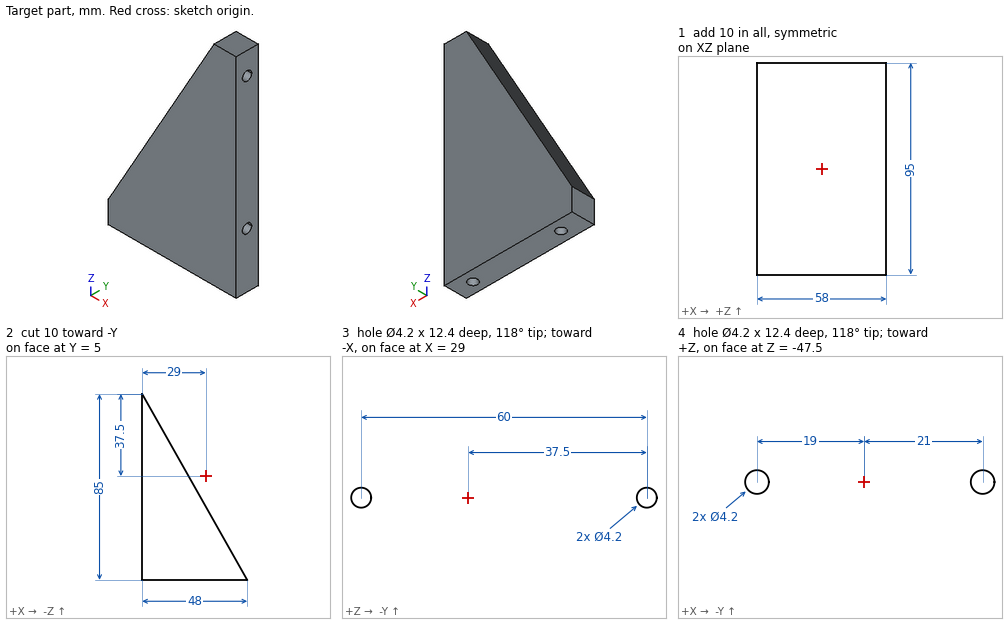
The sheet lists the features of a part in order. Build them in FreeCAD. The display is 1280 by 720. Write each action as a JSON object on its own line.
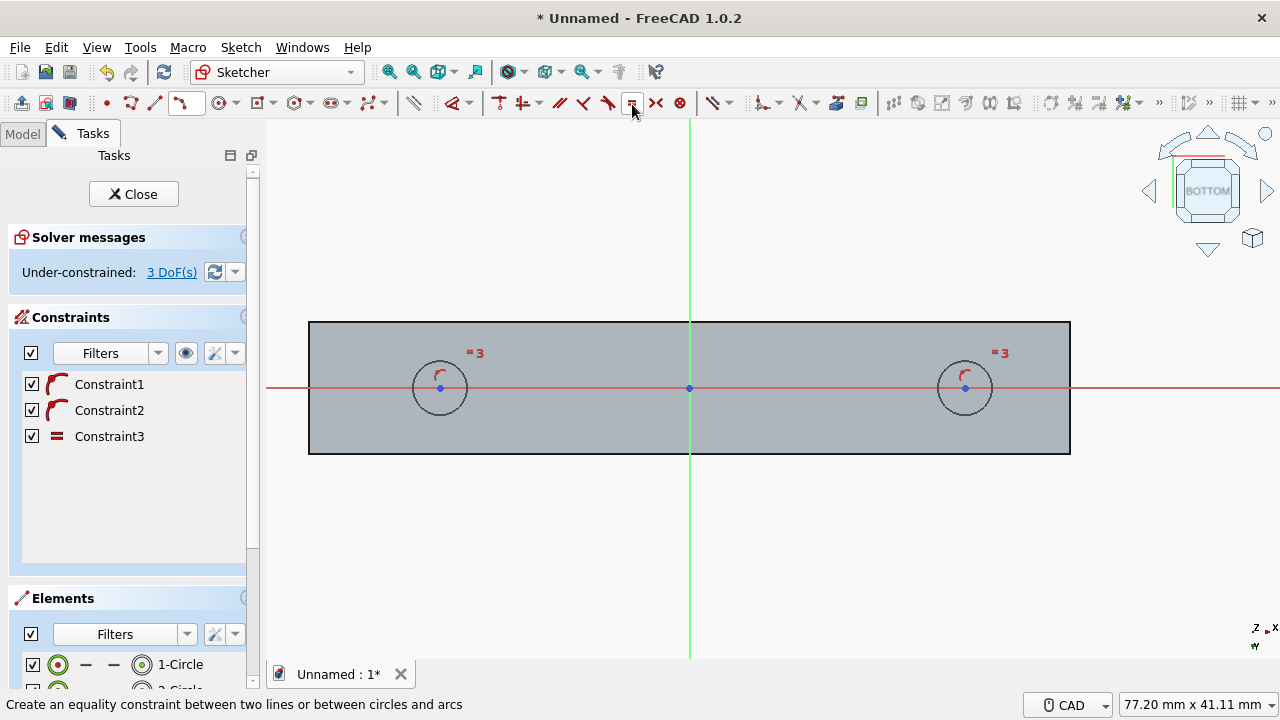
{"action": "left_click", "coordinate": [452, 104]}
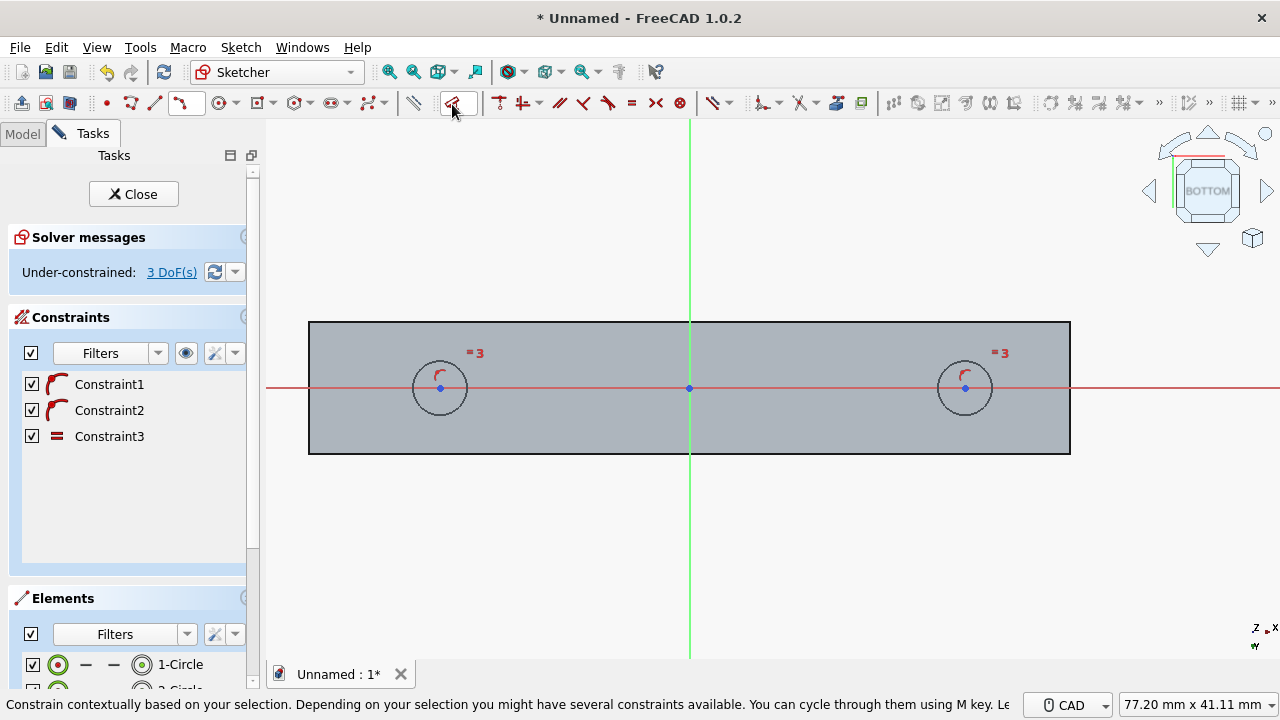
{"action": "left_click", "coordinate": [459, 369]}
{"action": "left_click", "coordinate": [482, 346]}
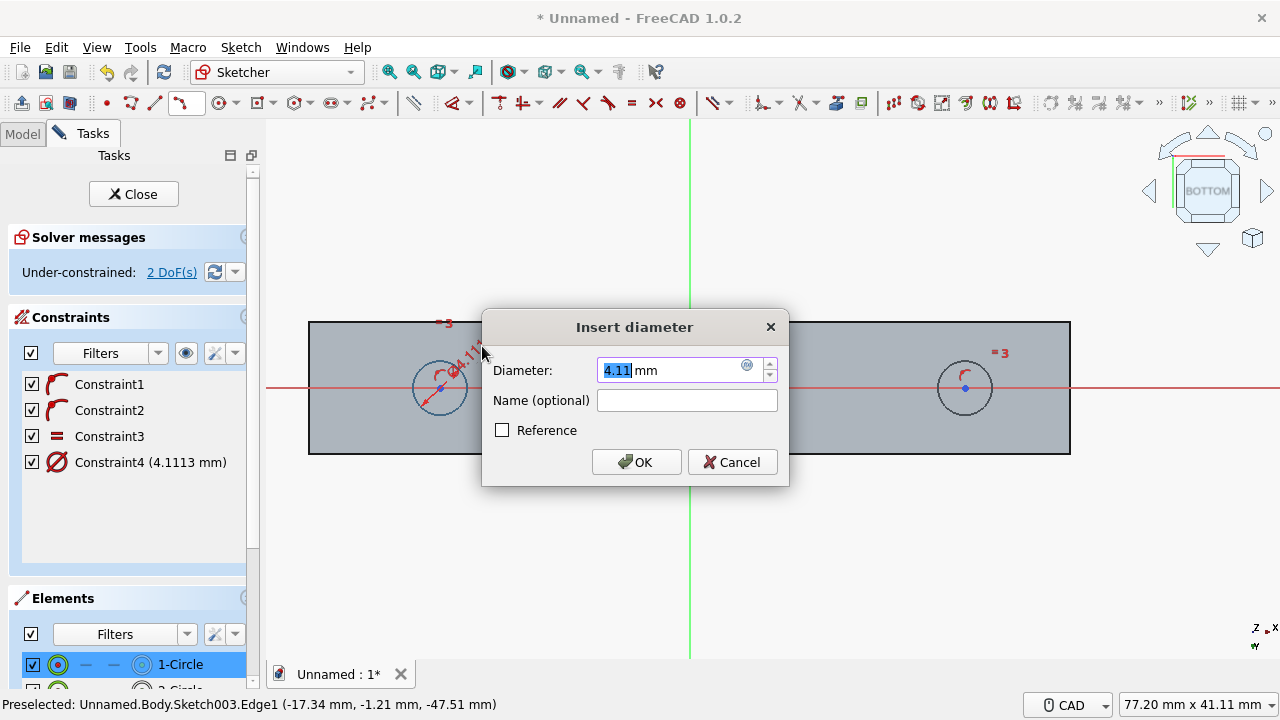
{"action": "type", "text": "4.2"}
{"action": "key", "text": "Return"}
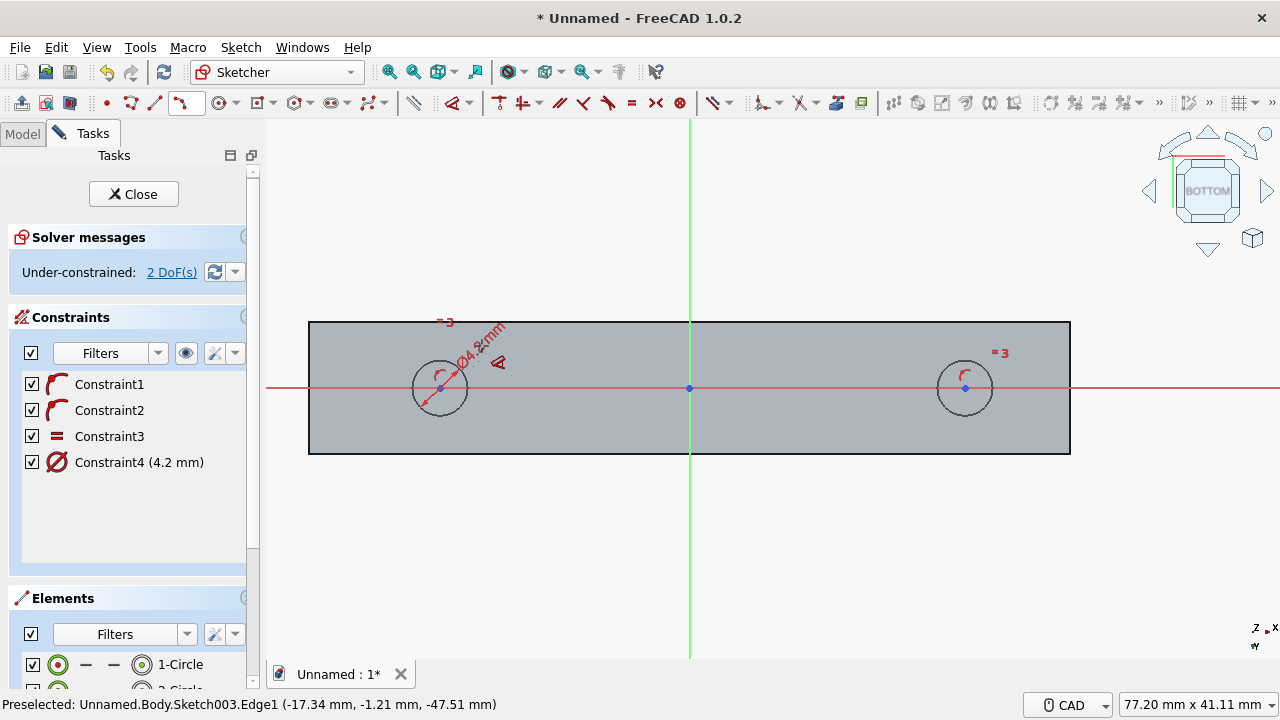
{"action": "left_click", "coordinate": [440, 388]}
{"action": "left_click", "coordinate": [565, 422]}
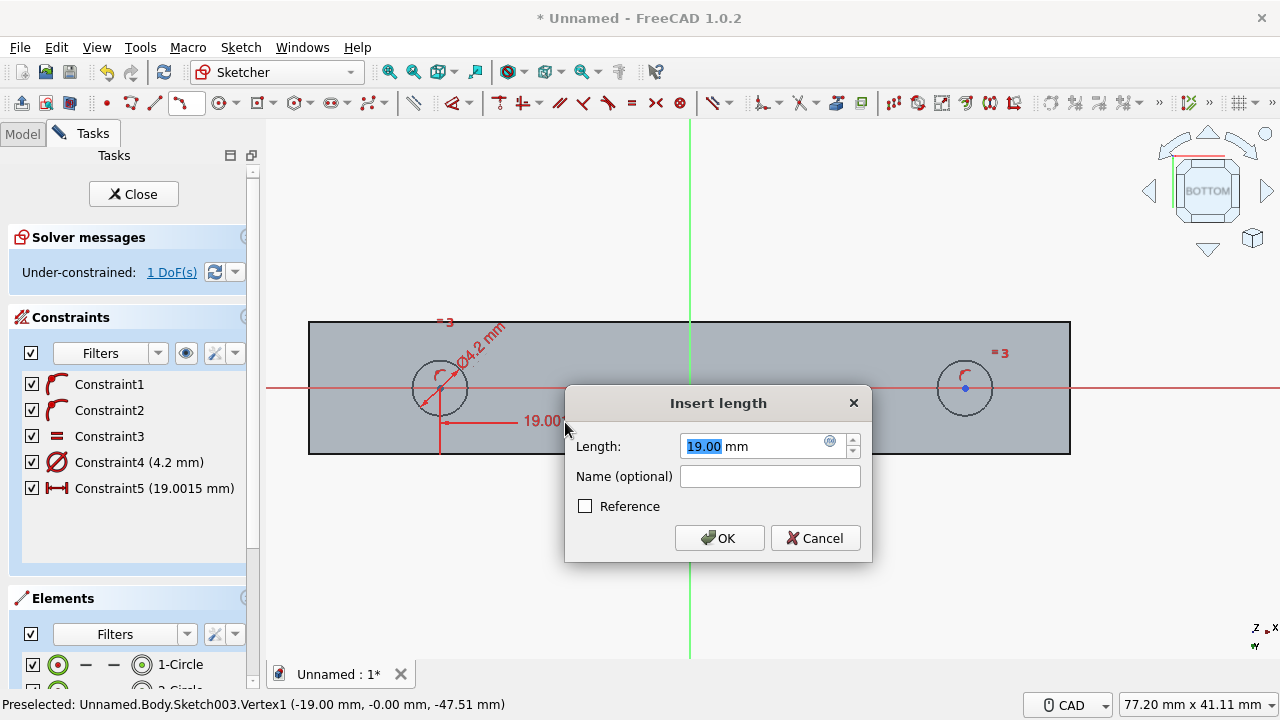
{"action": "type", "text": "19"}
{"action": "key", "text": "Return"}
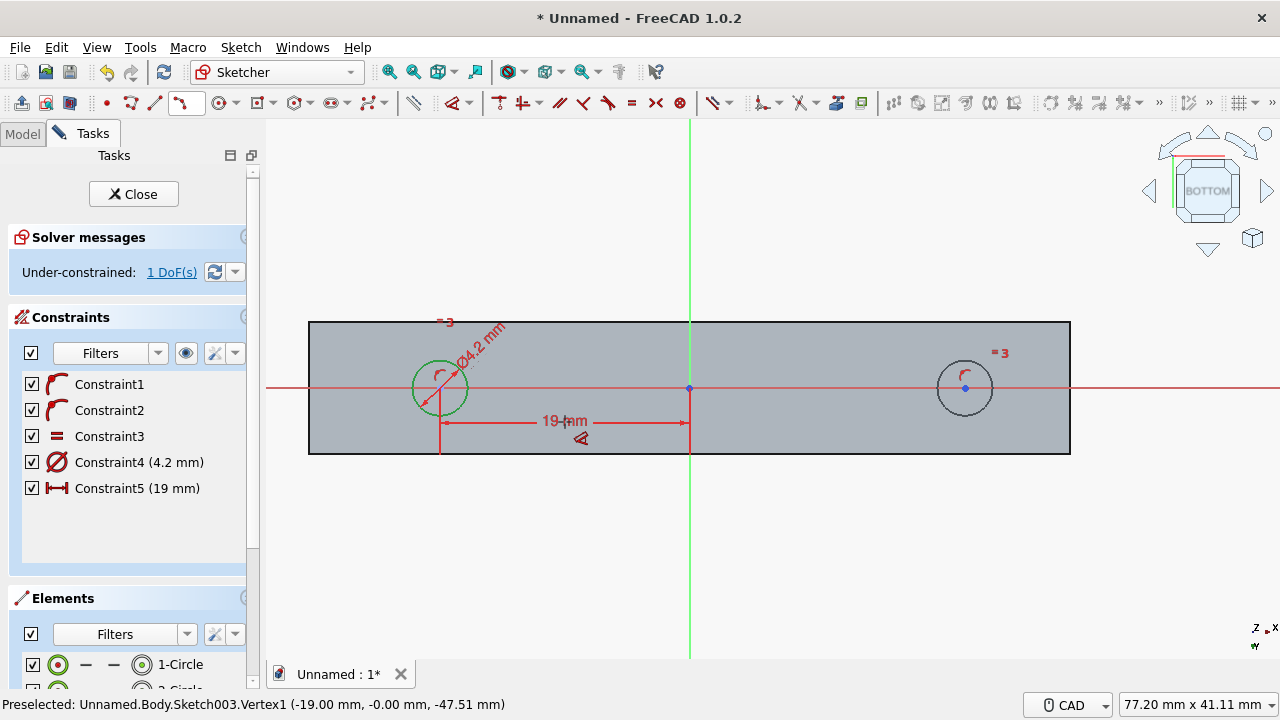
{"action": "left_click", "coordinate": [965, 388]}
{"action": "left_click", "coordinate": [827, 422]}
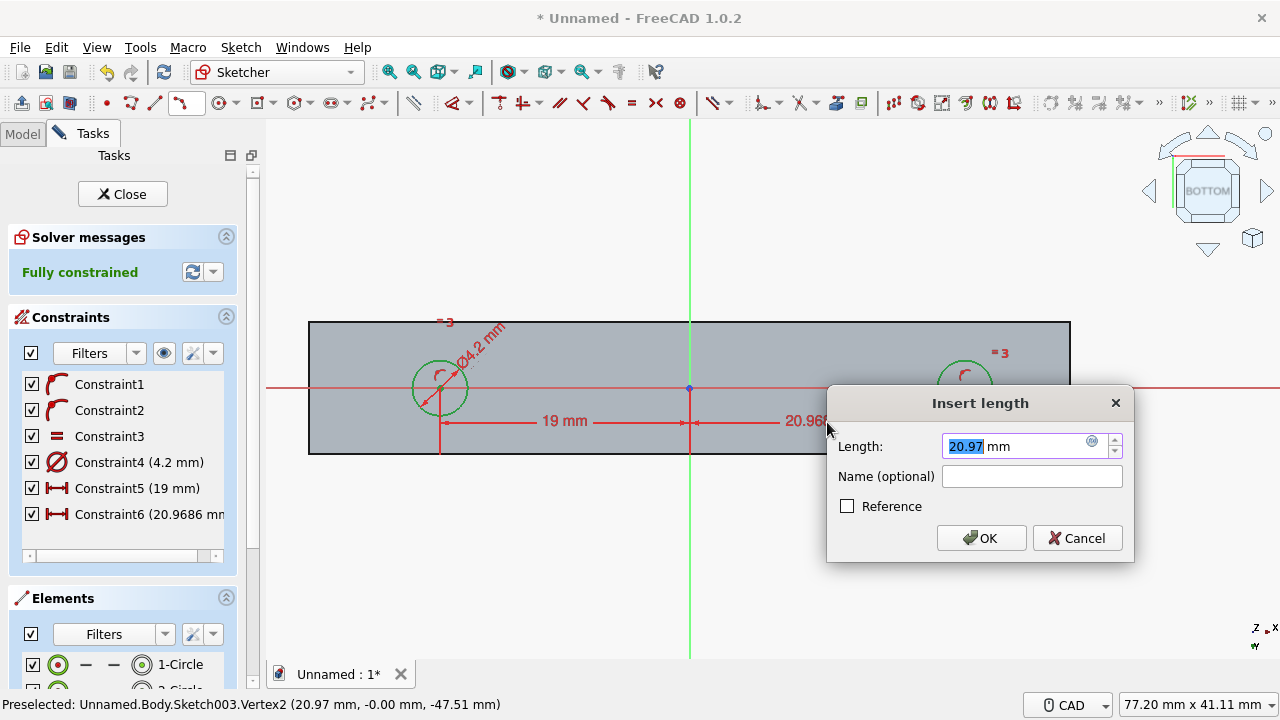
{"action": "type", "text": "21"}
{"action": "key", "text": "Return"}
{"action": "key", "text": "Escape"}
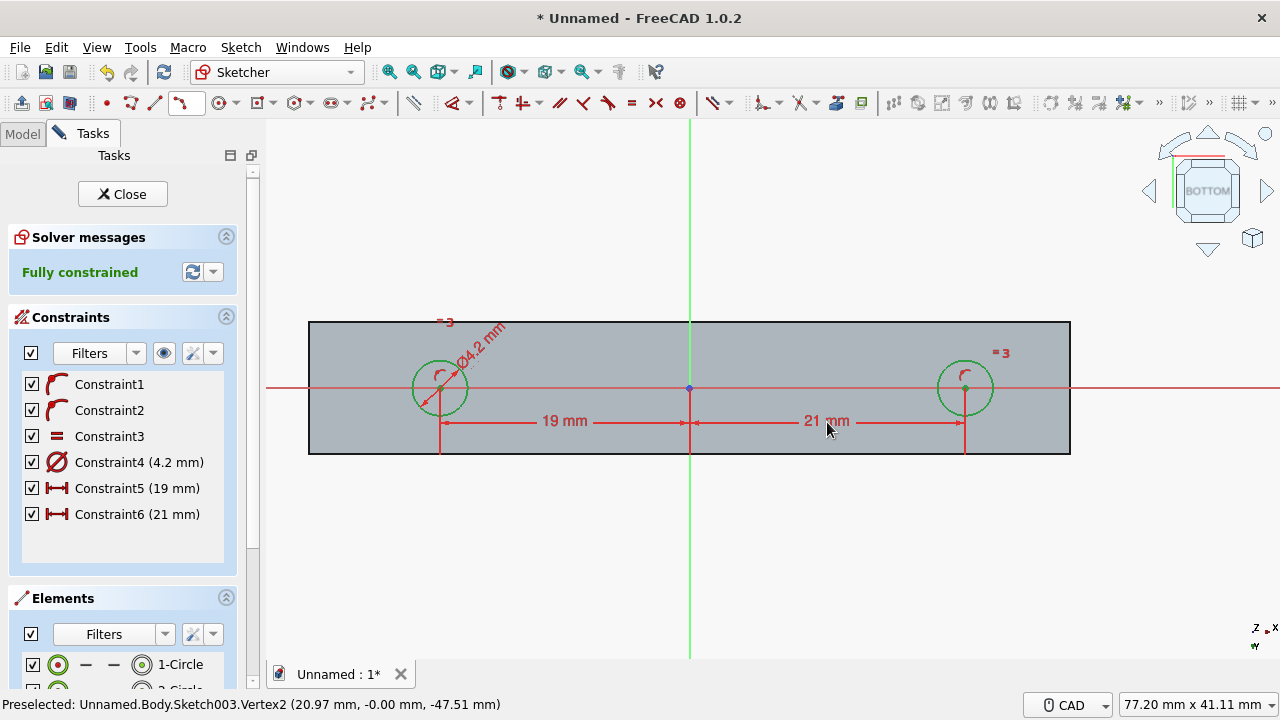
{"action": "left_click", "coordinate": [123, 194]}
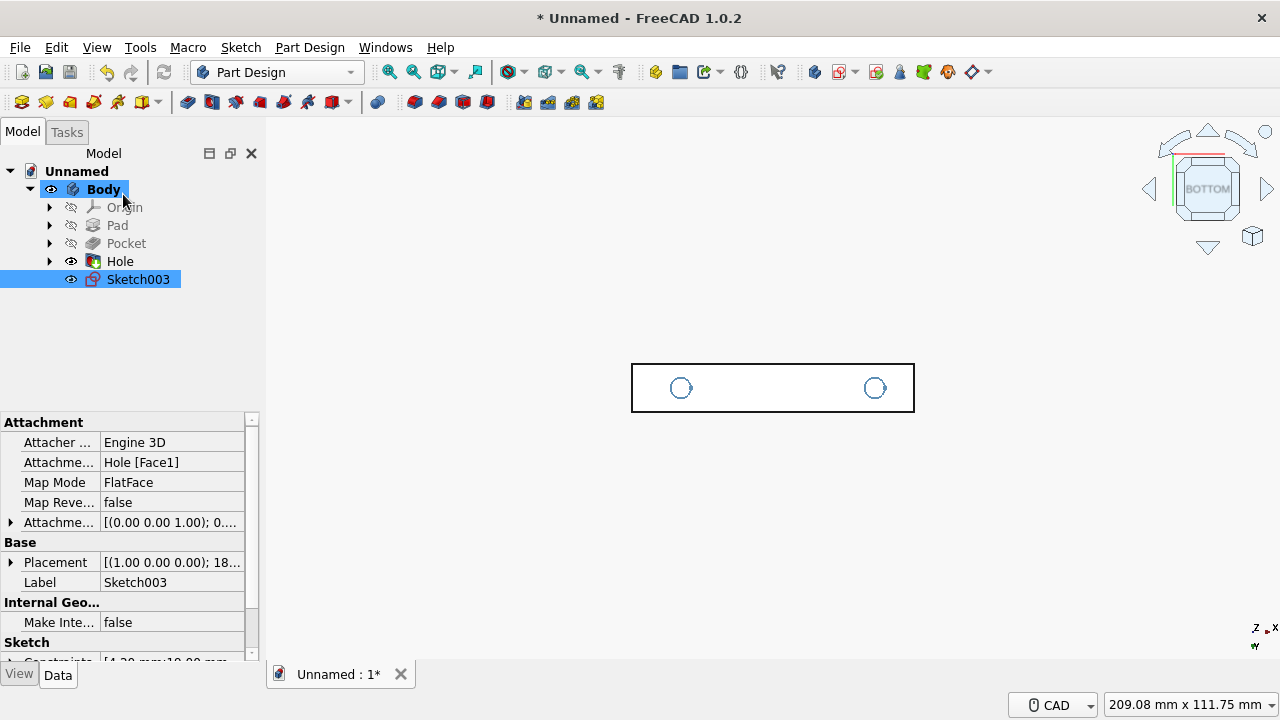
{"action": "left_click", "coordinate": [212, 102]}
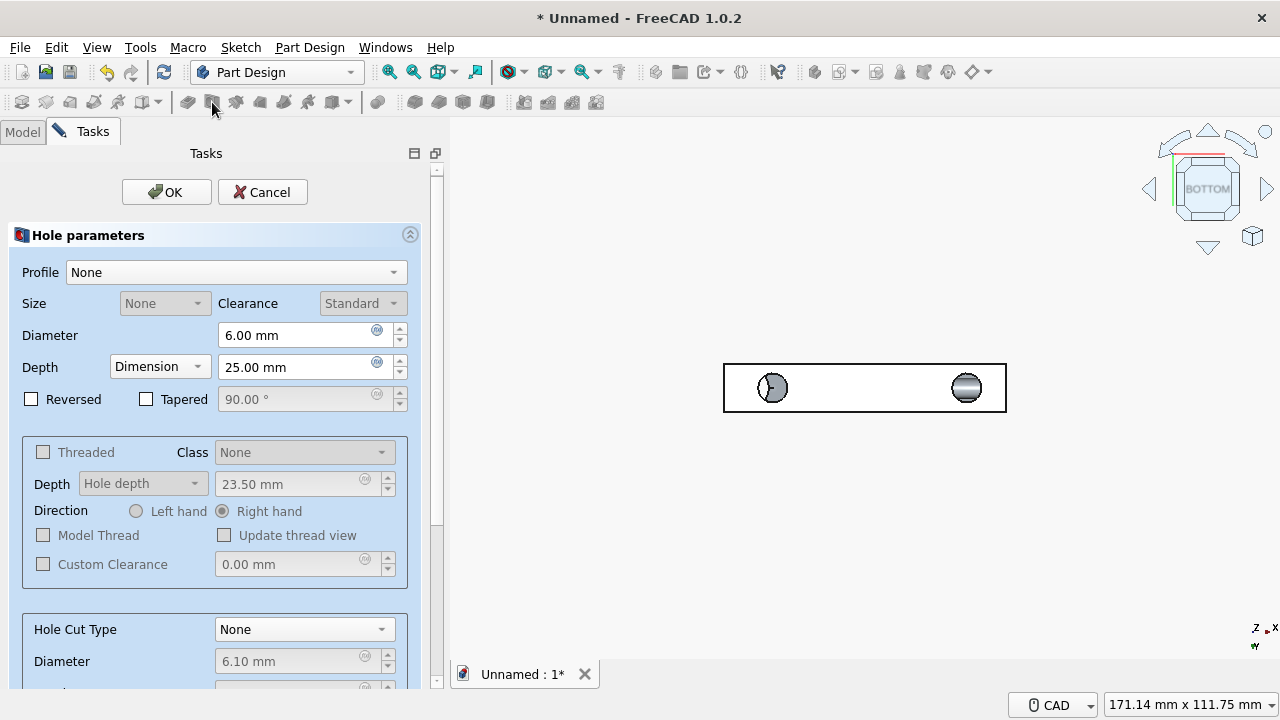
{"action": "triple_click", "coordinate": [305, 335]}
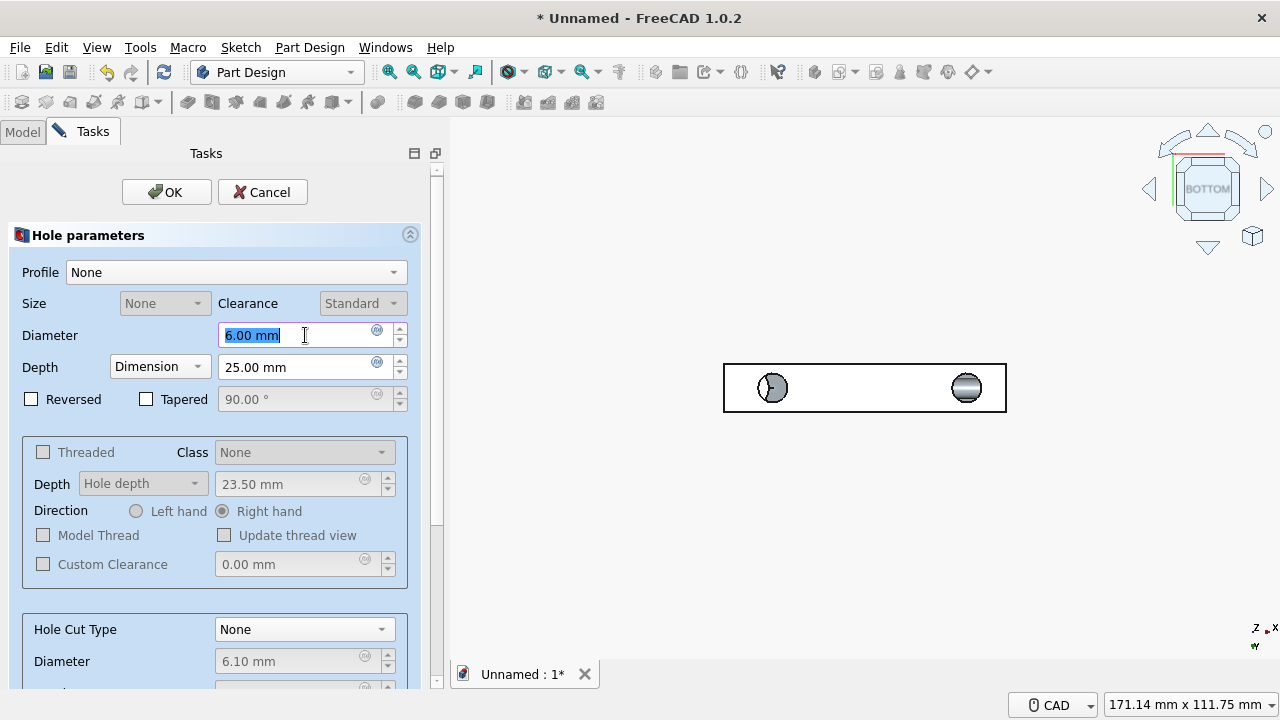
{"action": "type", "text": "4.2"}
{"action": "key", "text": "Tab"}